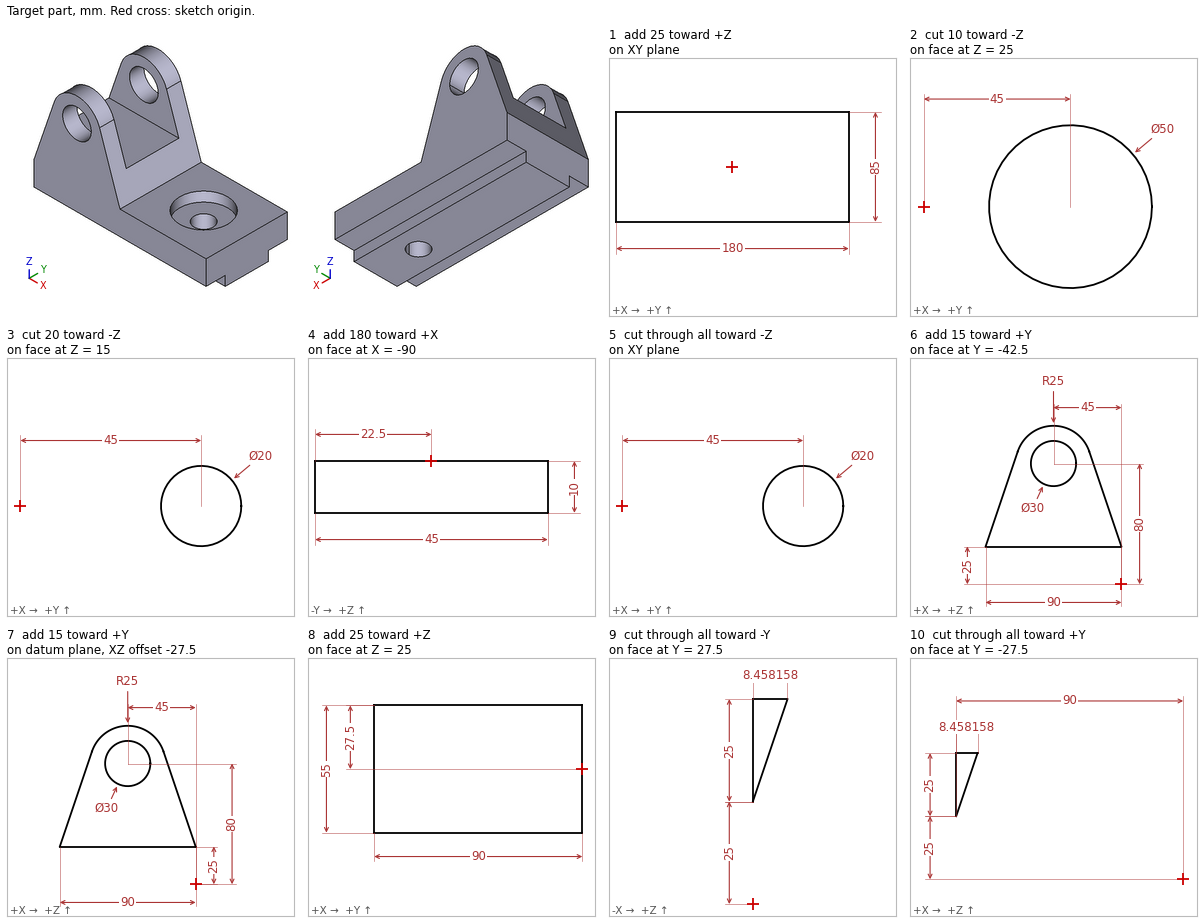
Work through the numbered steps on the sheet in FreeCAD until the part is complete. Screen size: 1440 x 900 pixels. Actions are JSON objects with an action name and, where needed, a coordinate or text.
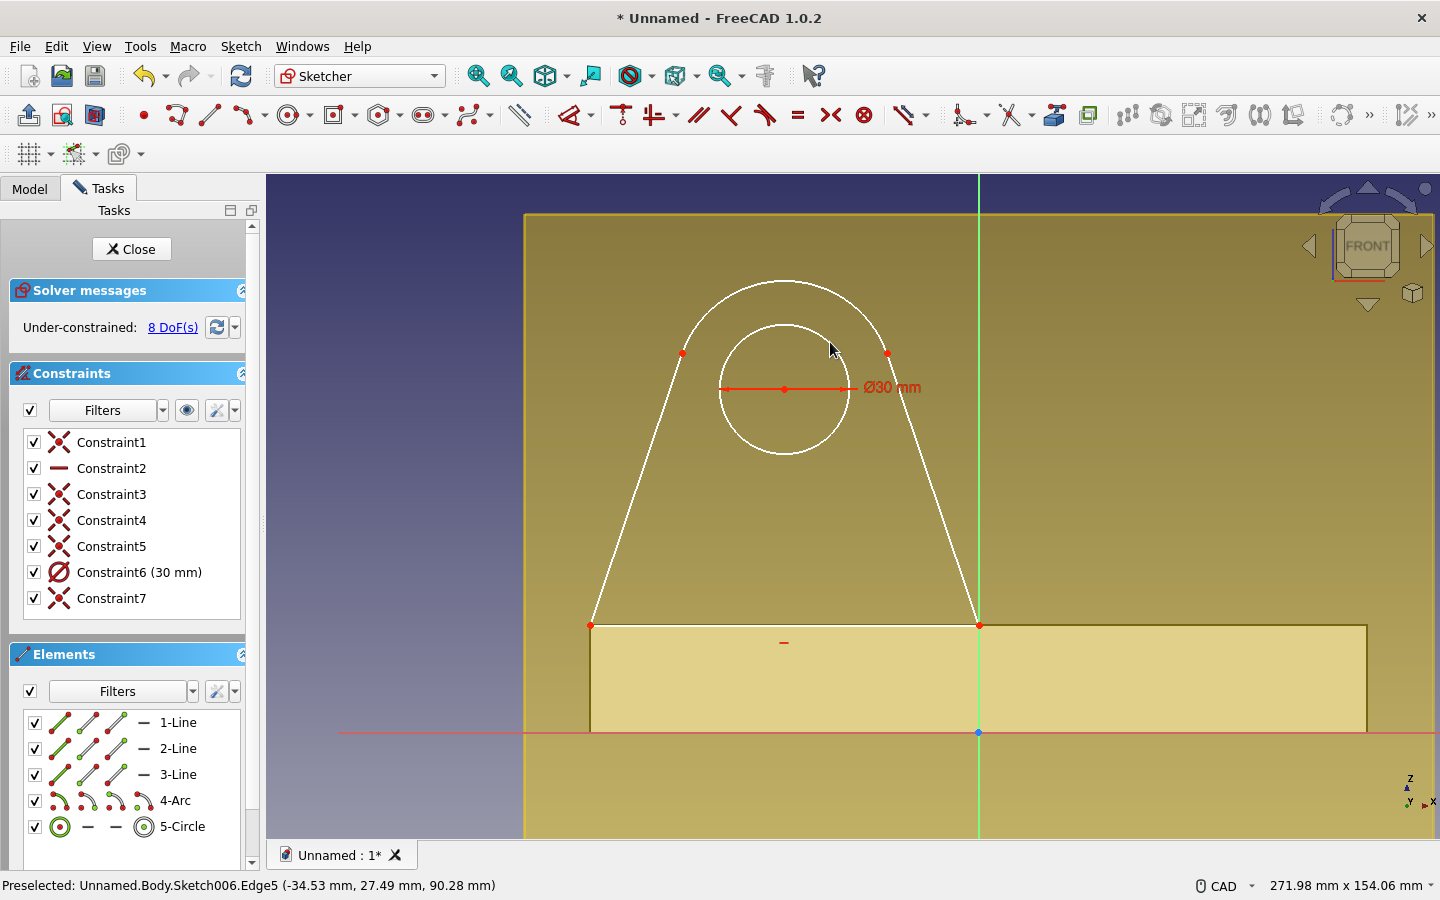
{"action": "left_click", "coordinate": [915, 436]}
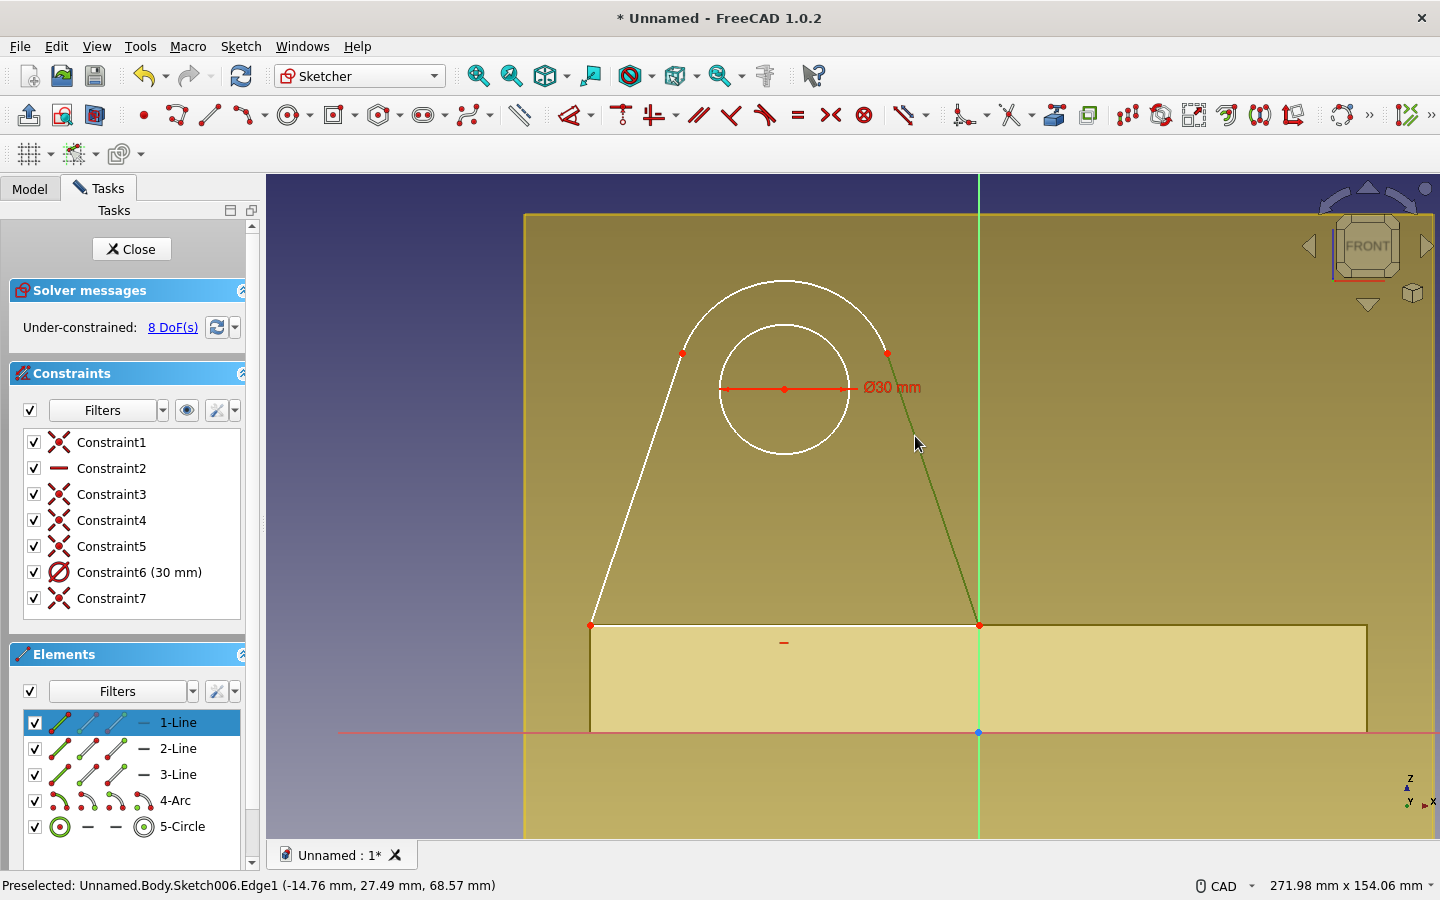
{"action": "left_click", "coordinate": [836, 294]}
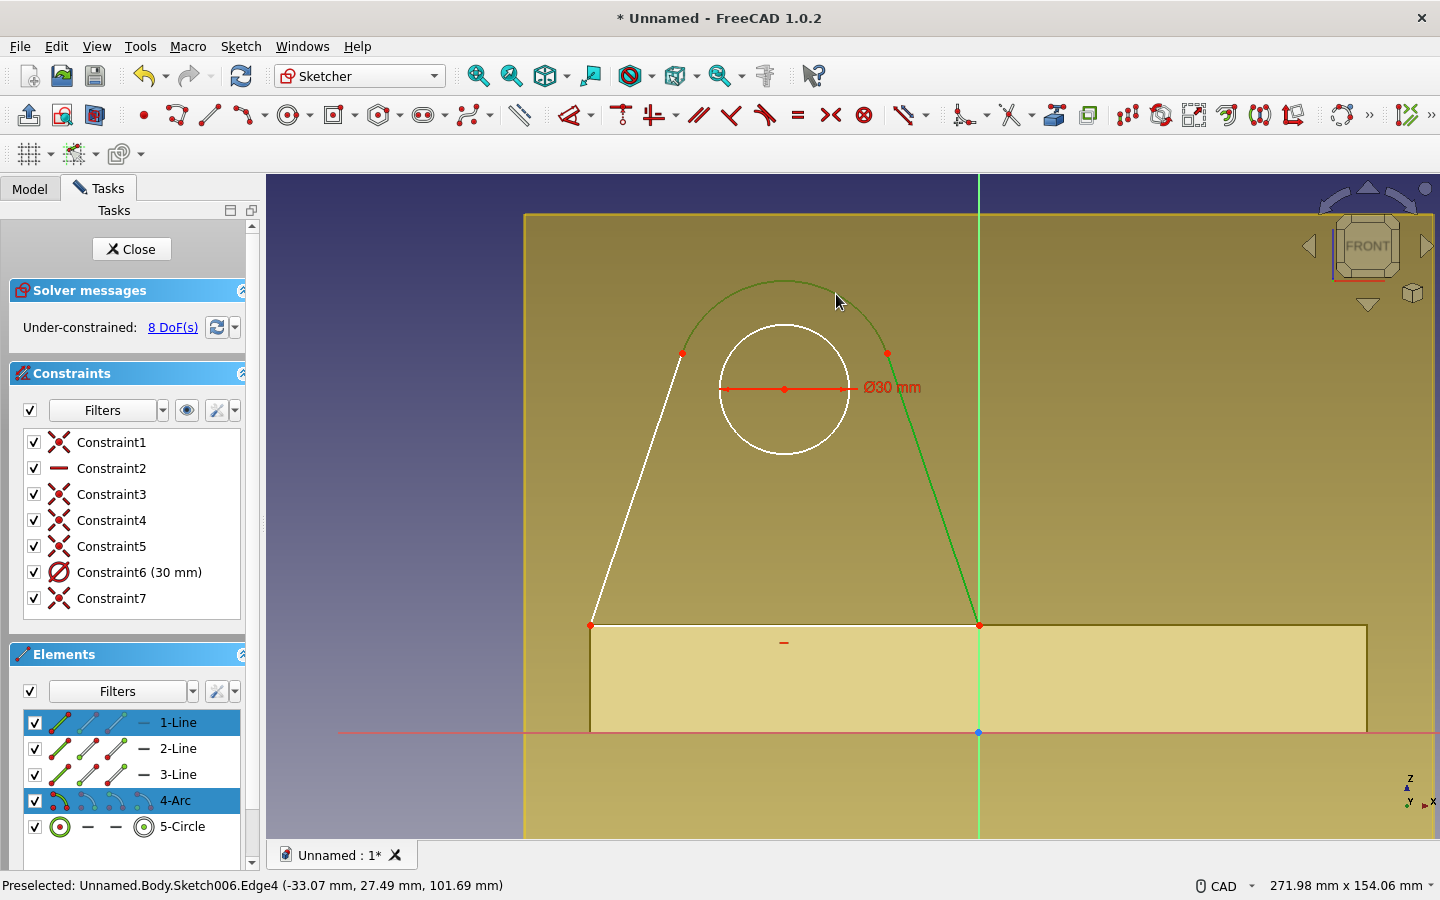
{"action": "left_click", "coordinate": [765, 116]}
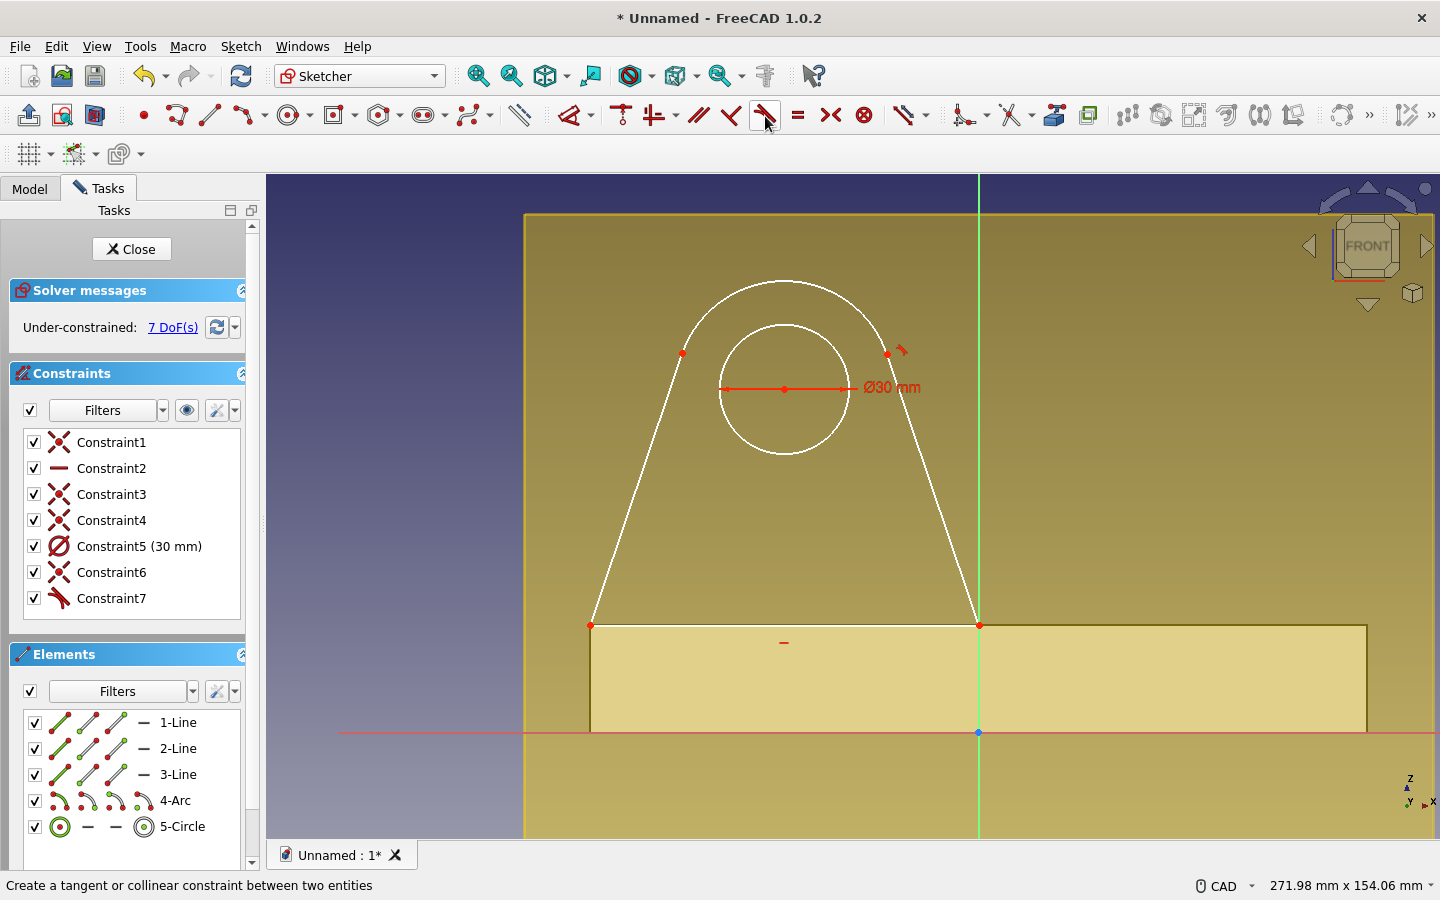
{"action": "left_click", "coordinate": [618, 544]}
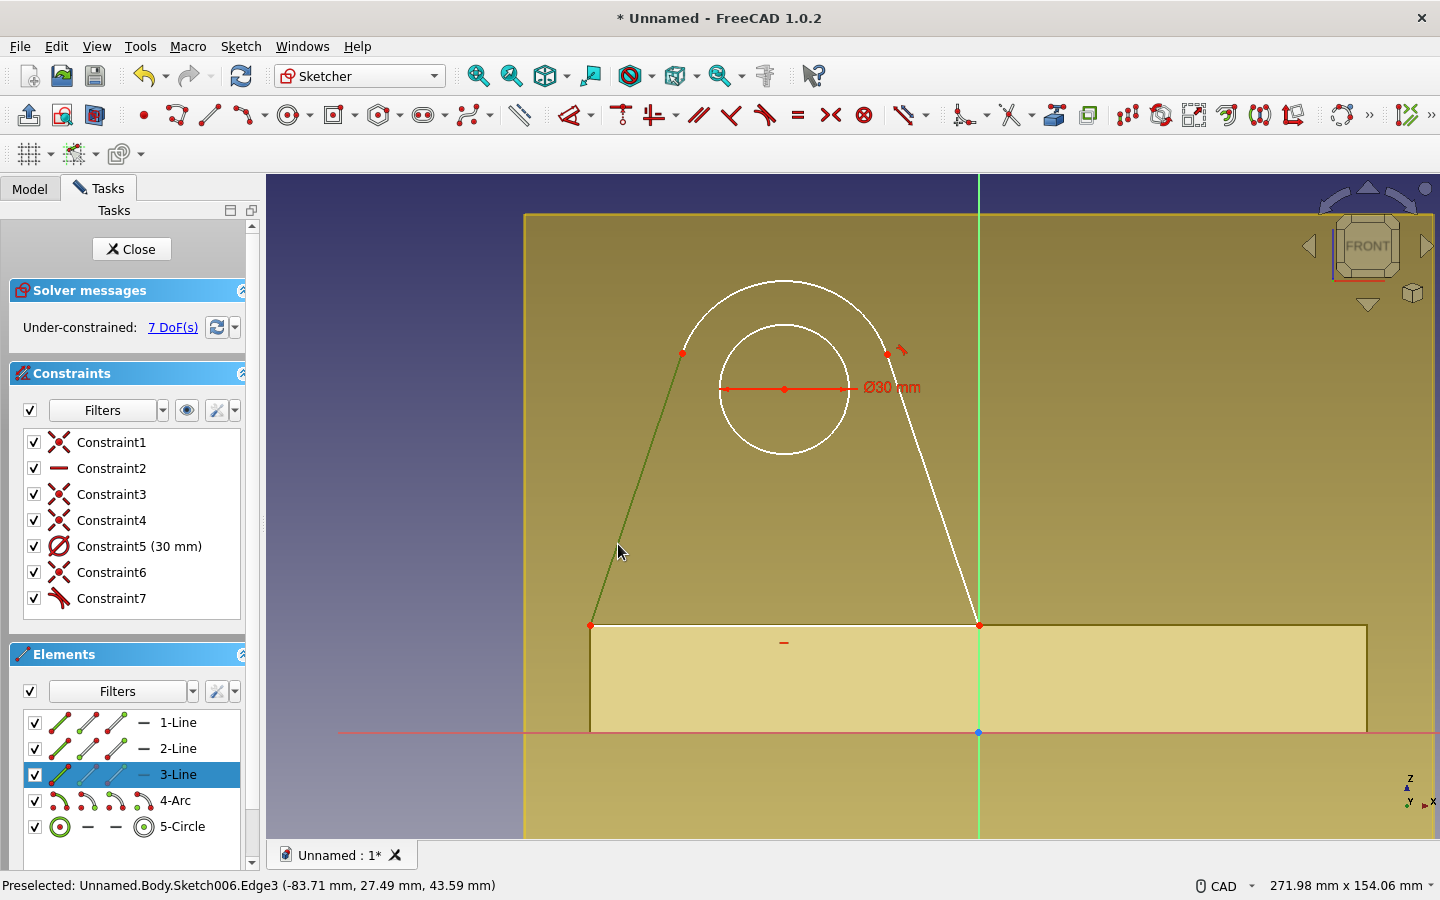
{"action": "left_click", "coordinate": [836, 294]}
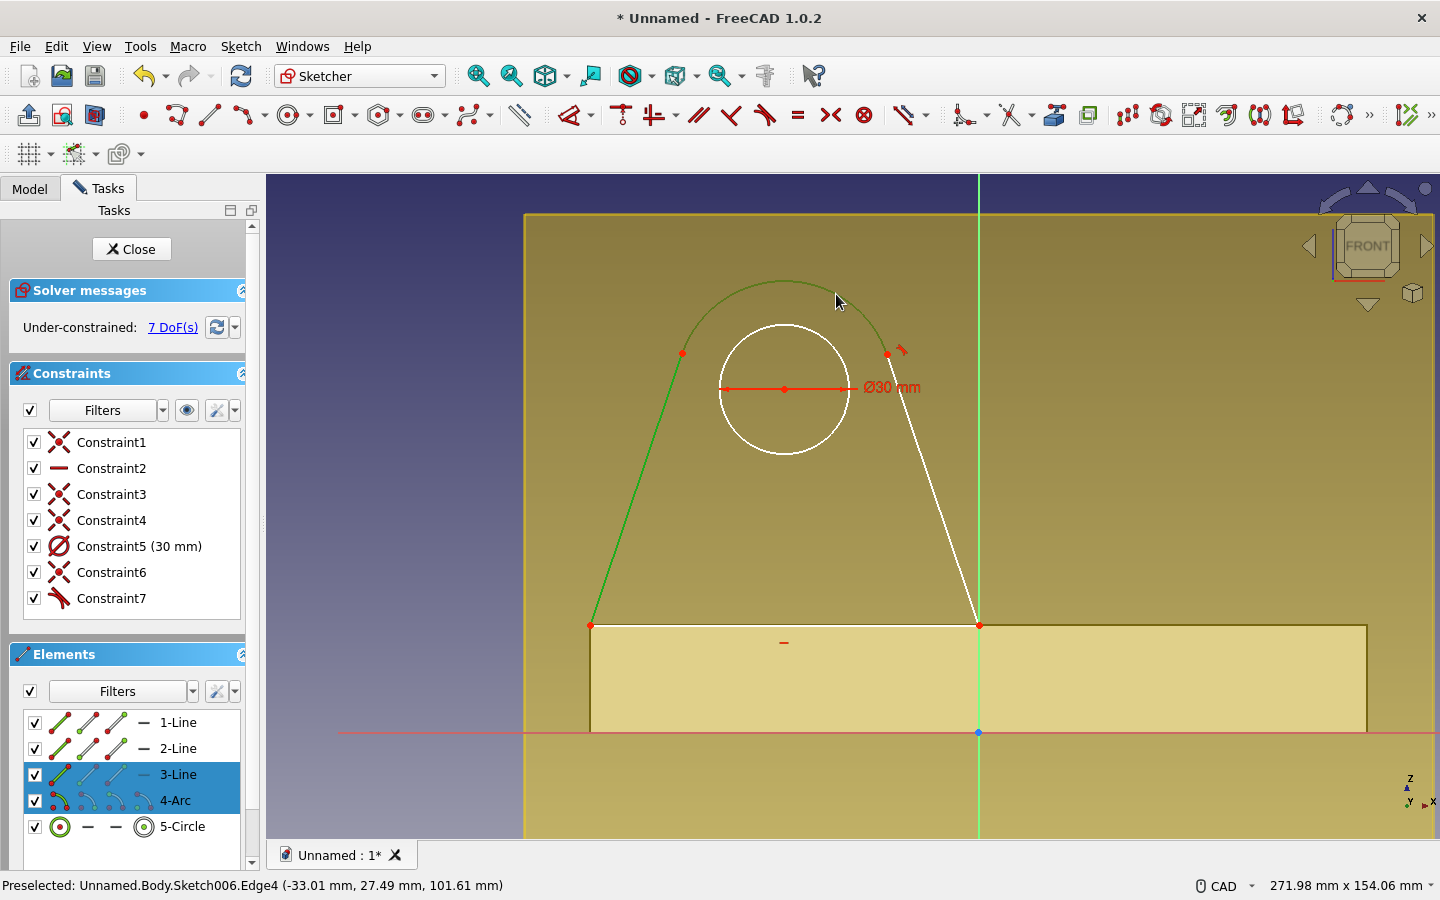
{"action": "left_click", "coordinate": [765, 116]}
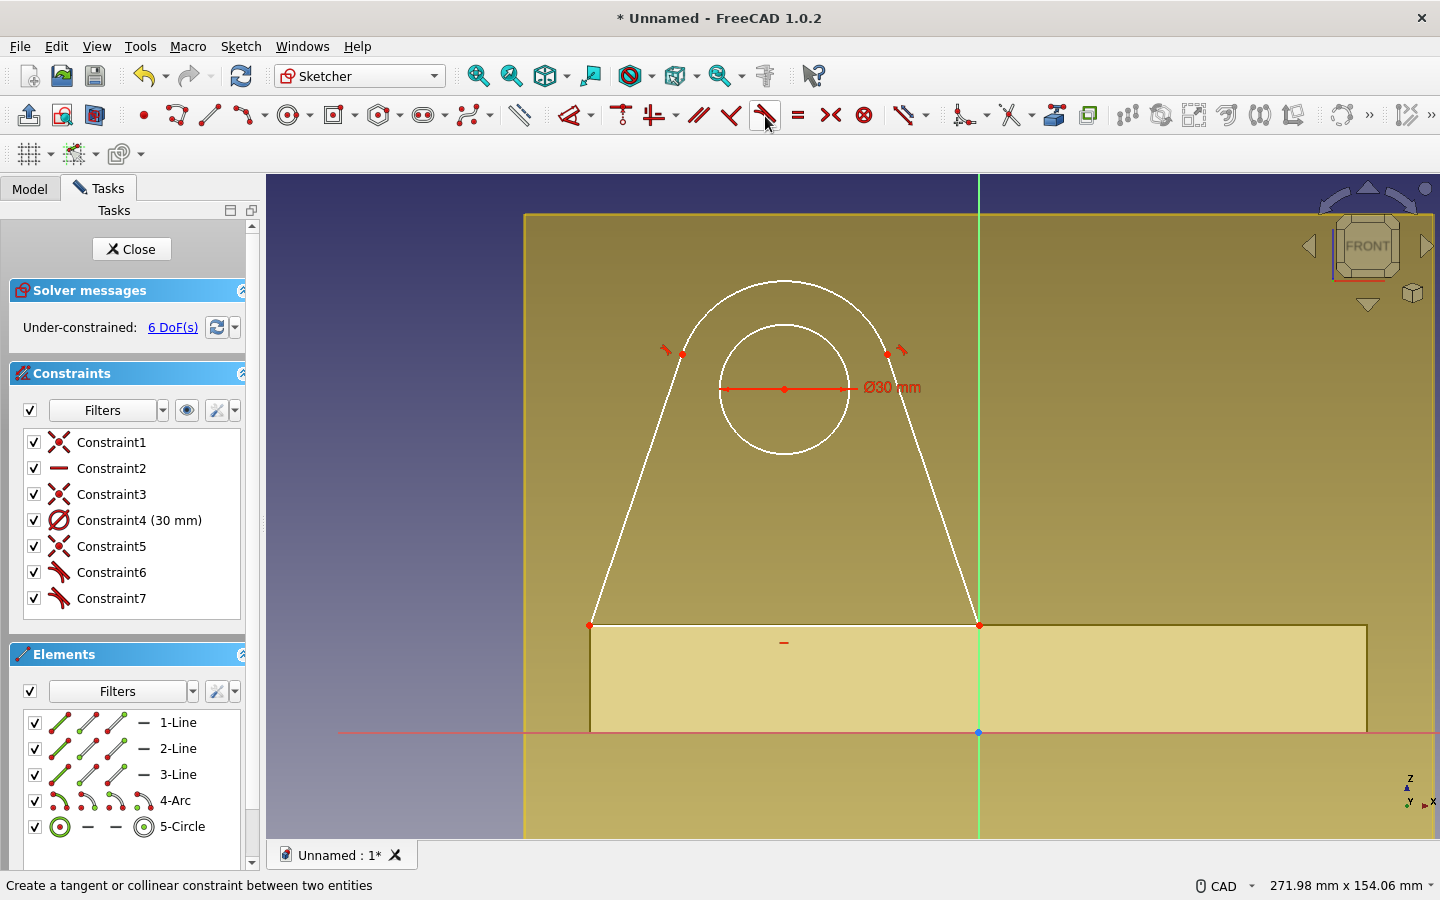
{"action": "left_click", "coordinate": [568, 116]}